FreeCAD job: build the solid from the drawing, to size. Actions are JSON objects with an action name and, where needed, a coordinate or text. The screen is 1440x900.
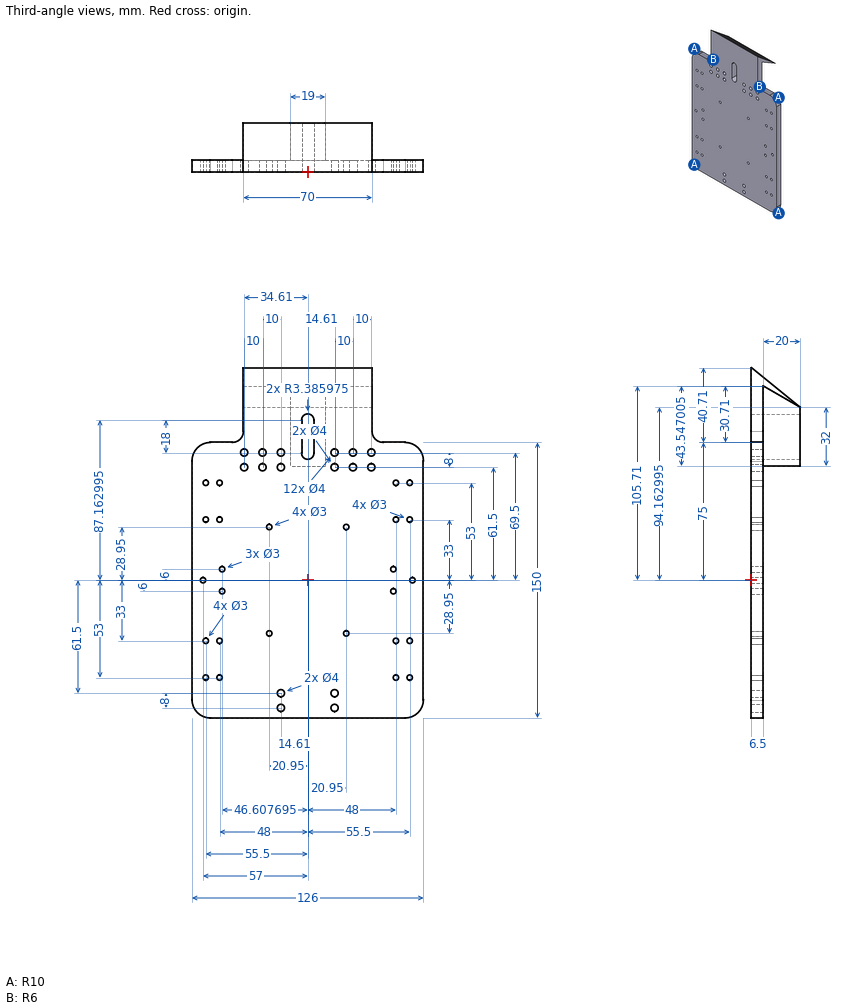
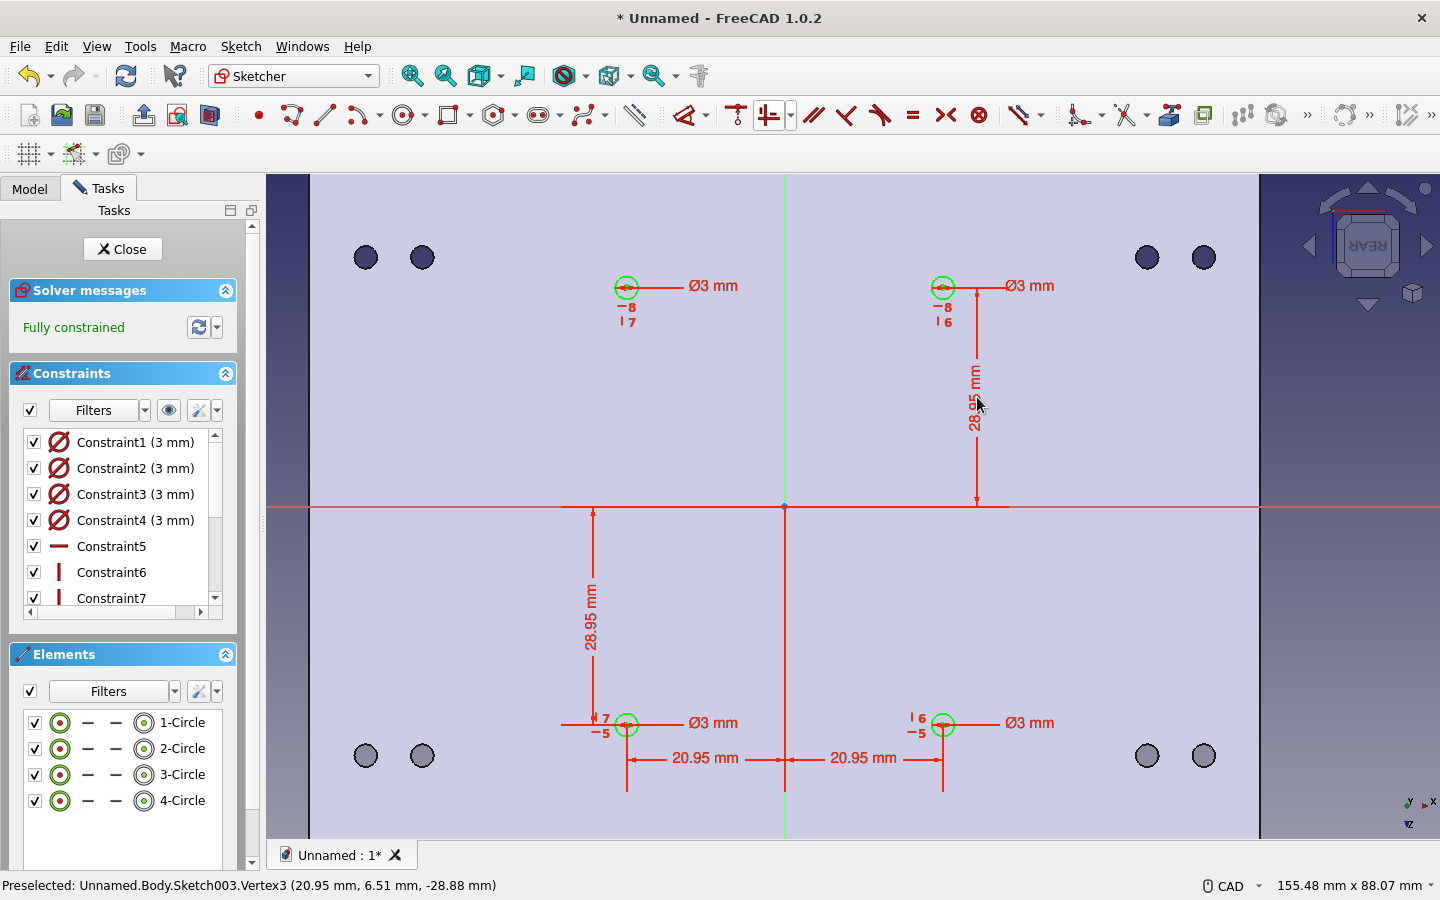
{"action": "left_click", "coordinate": [123, 249]}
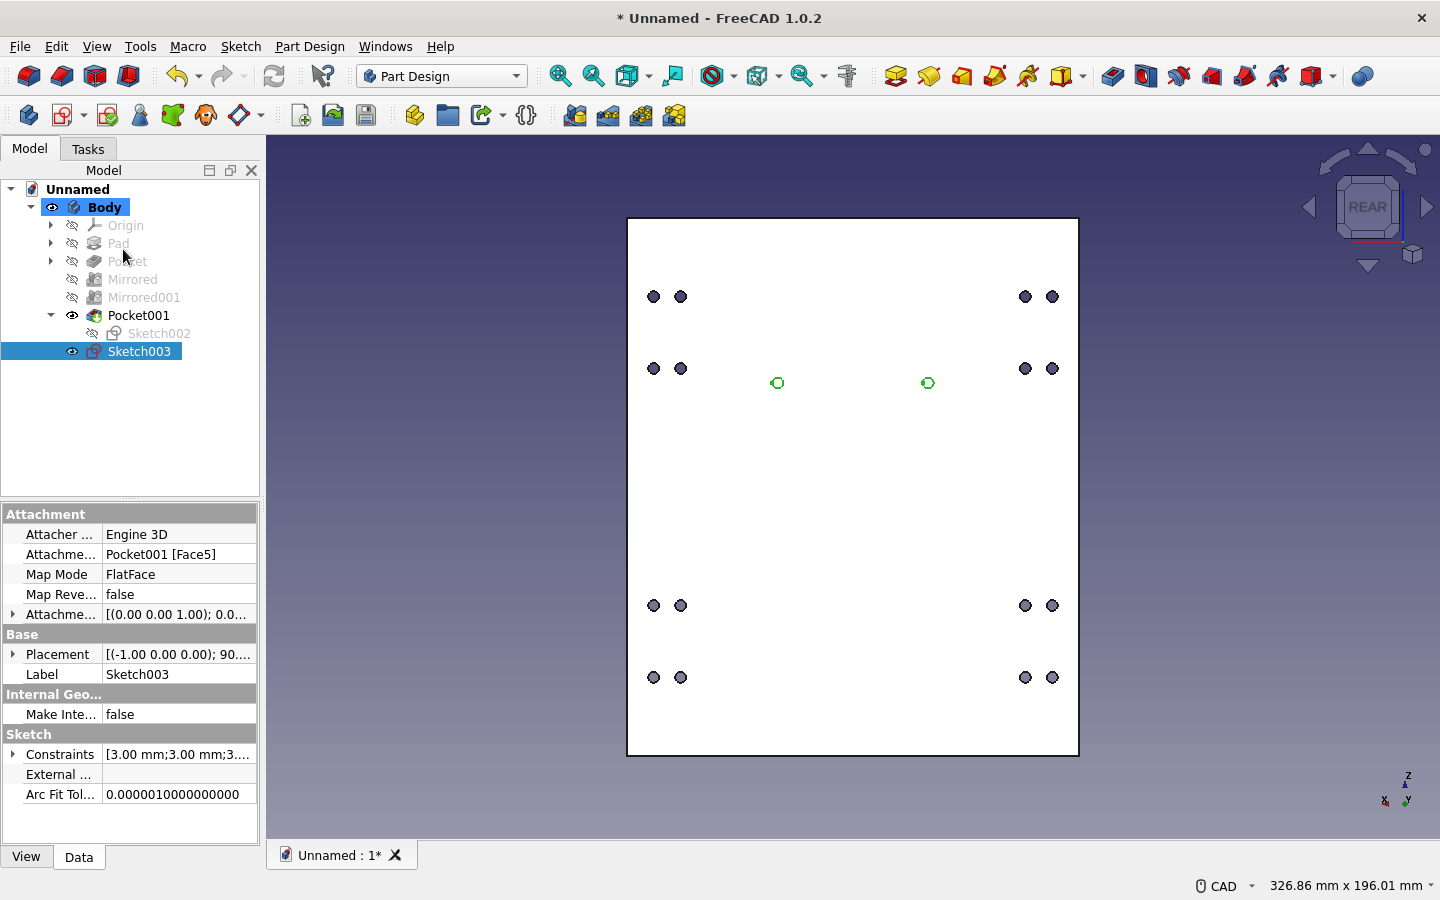
{"action": "left_click", "coordinate": [1113, 76]}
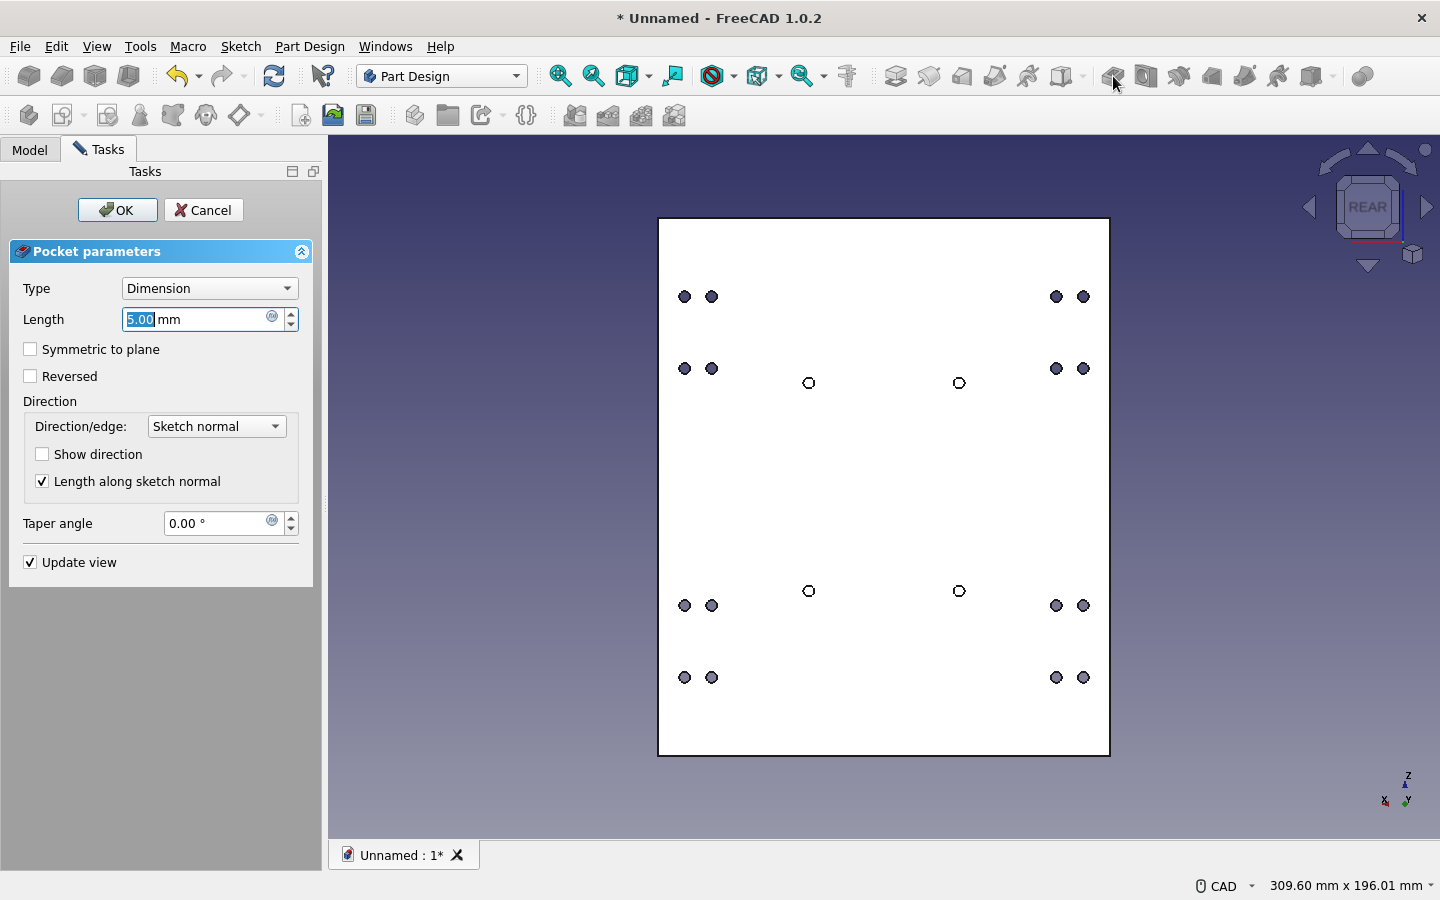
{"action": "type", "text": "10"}
{"action": "key", "text": "Tab"}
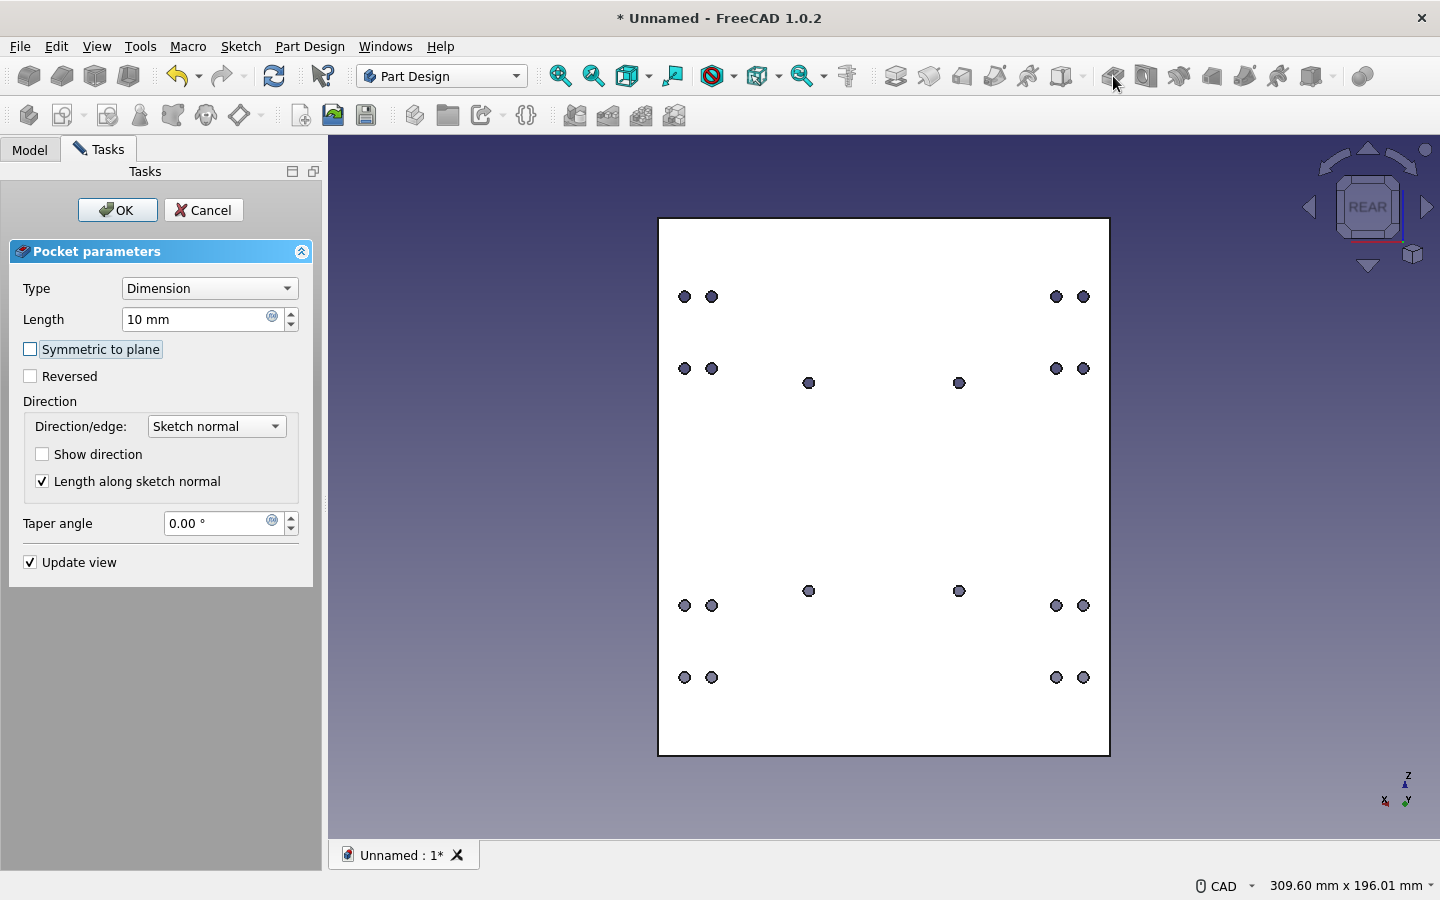
{"action": "left_click", "coordinate": [118, 210]}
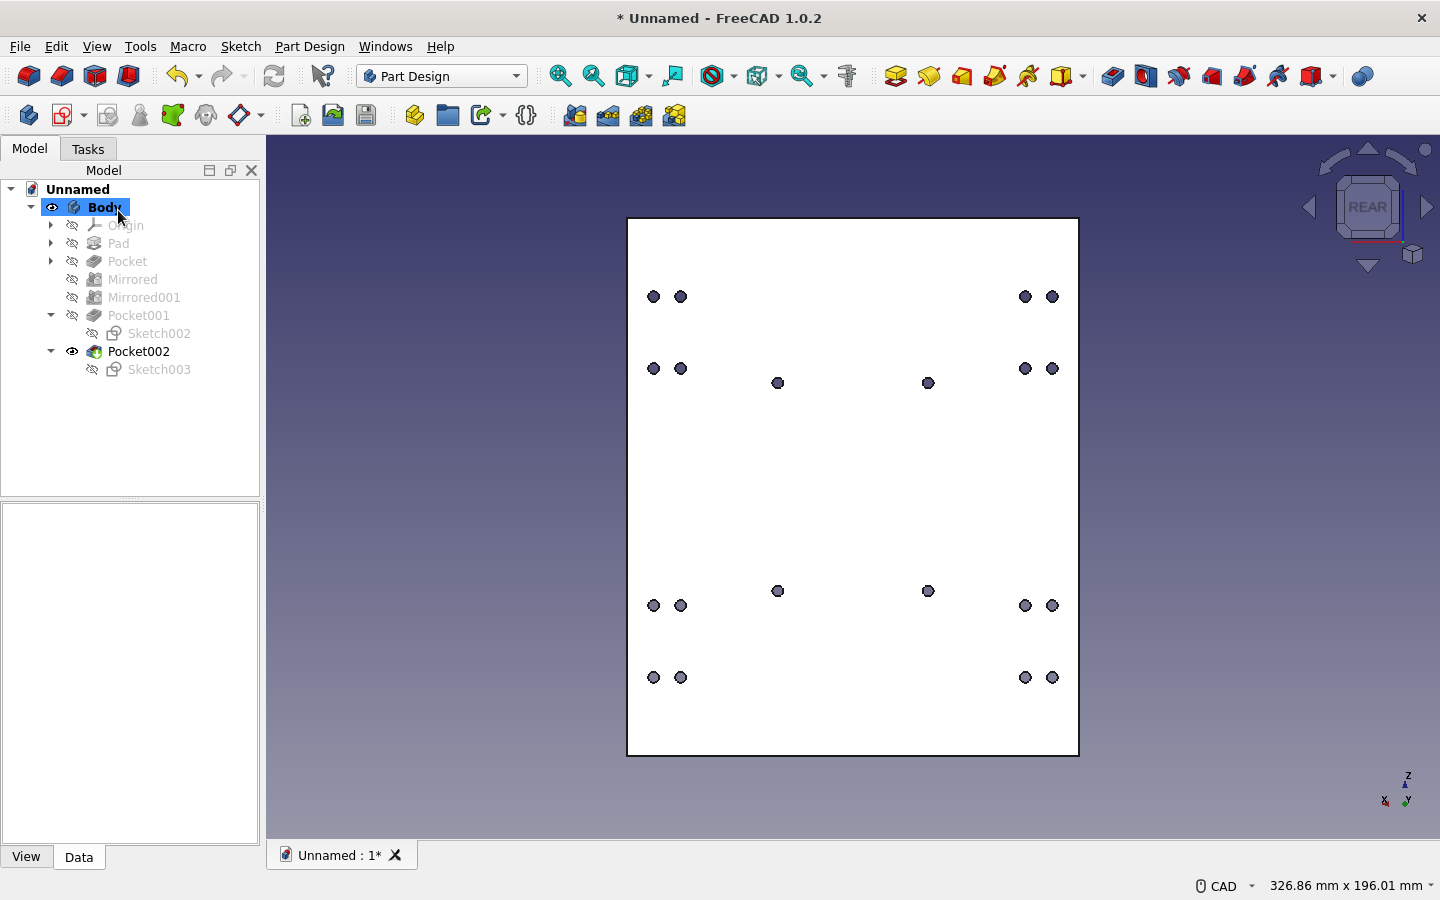
{"action": "key", "text": "0"}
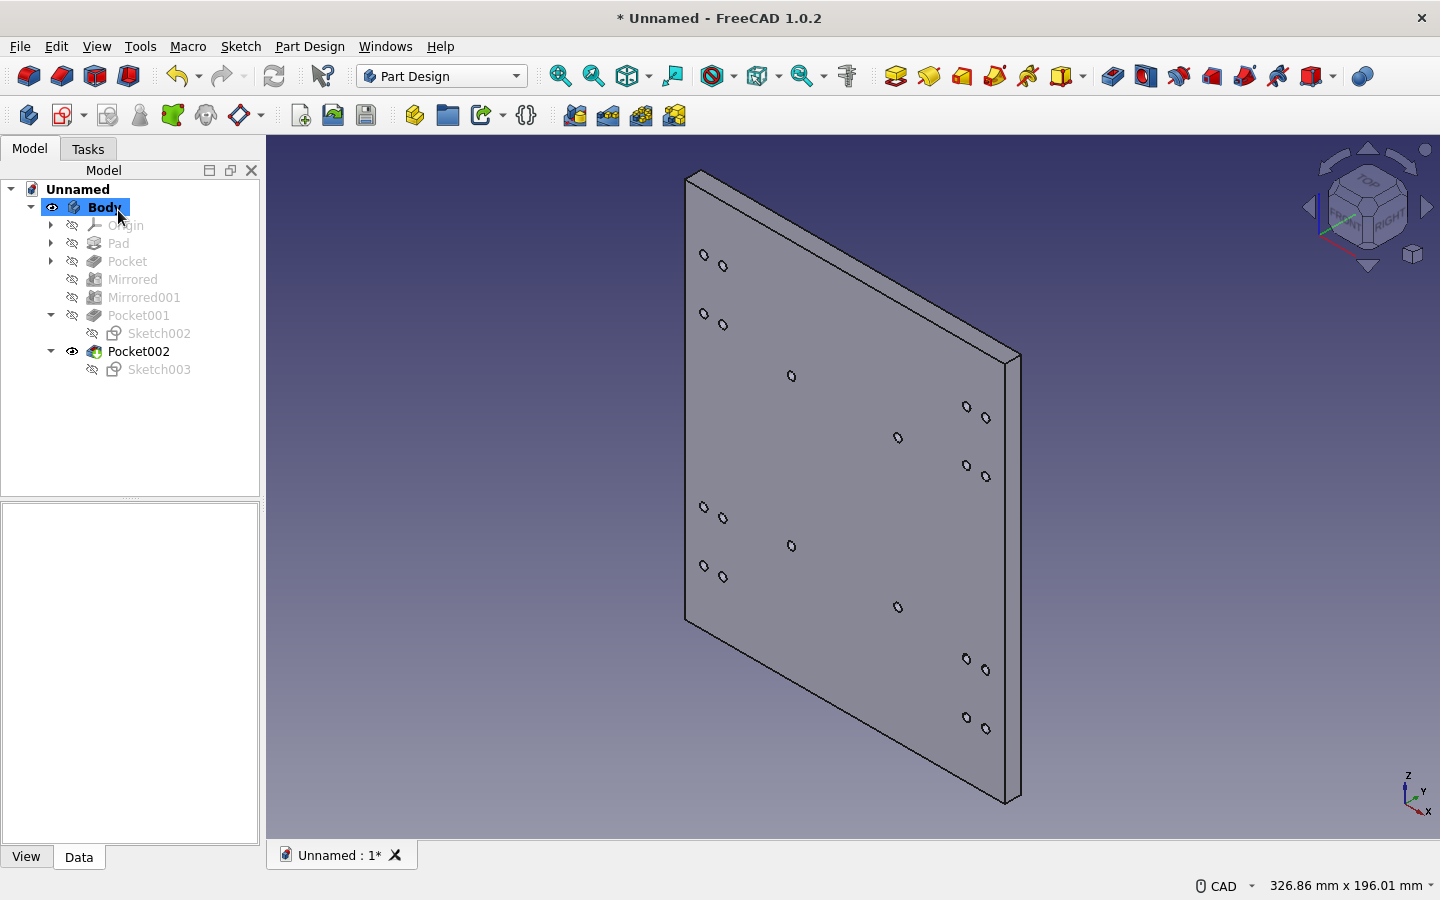
{"action": "left_click", "coordinate": [1013, 358]}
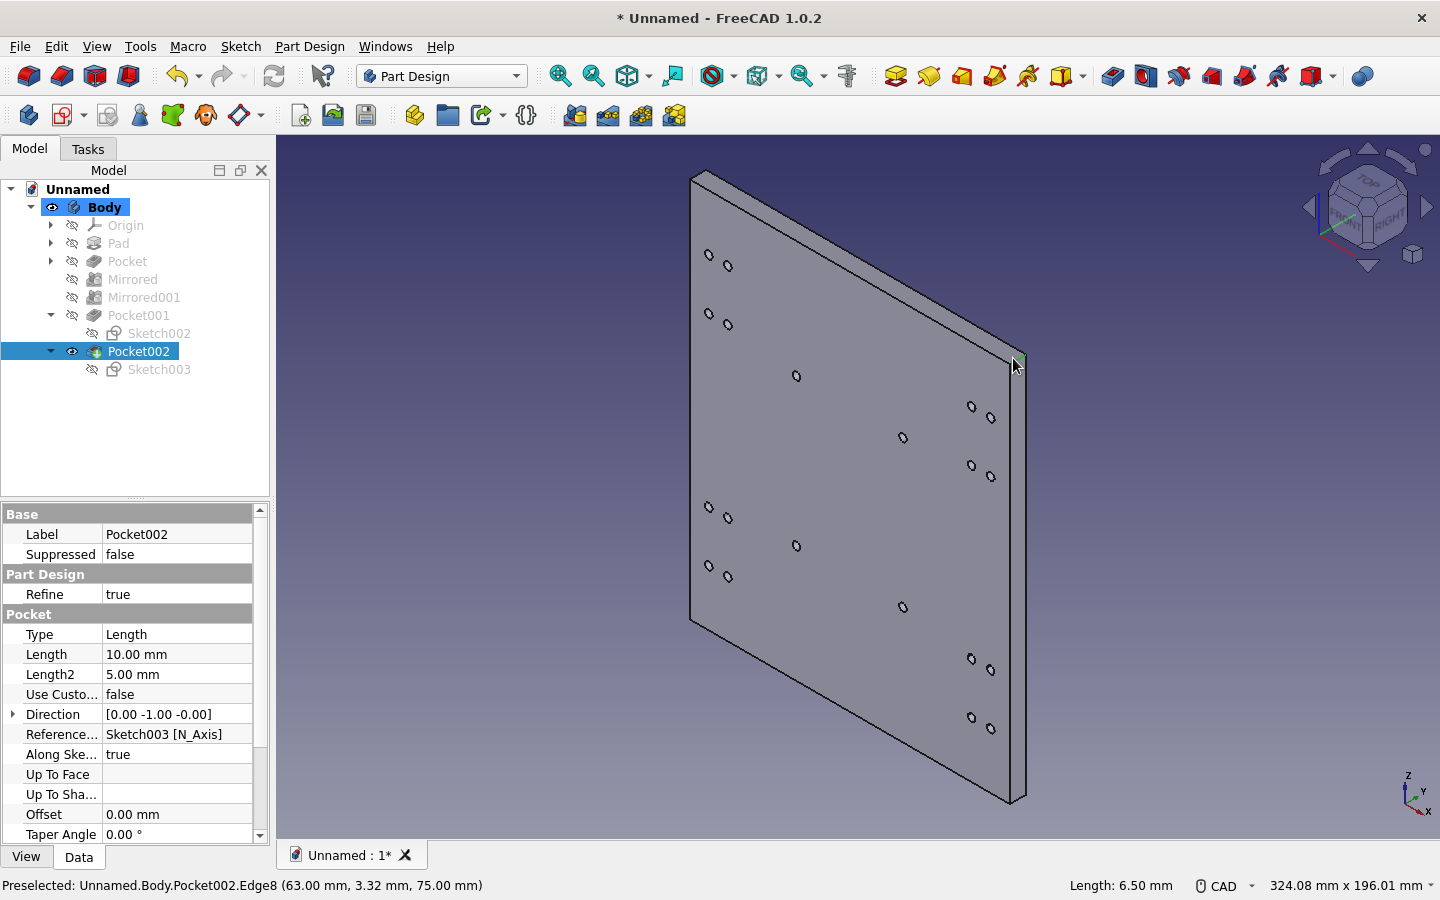
{"action": "key", "text": "2"}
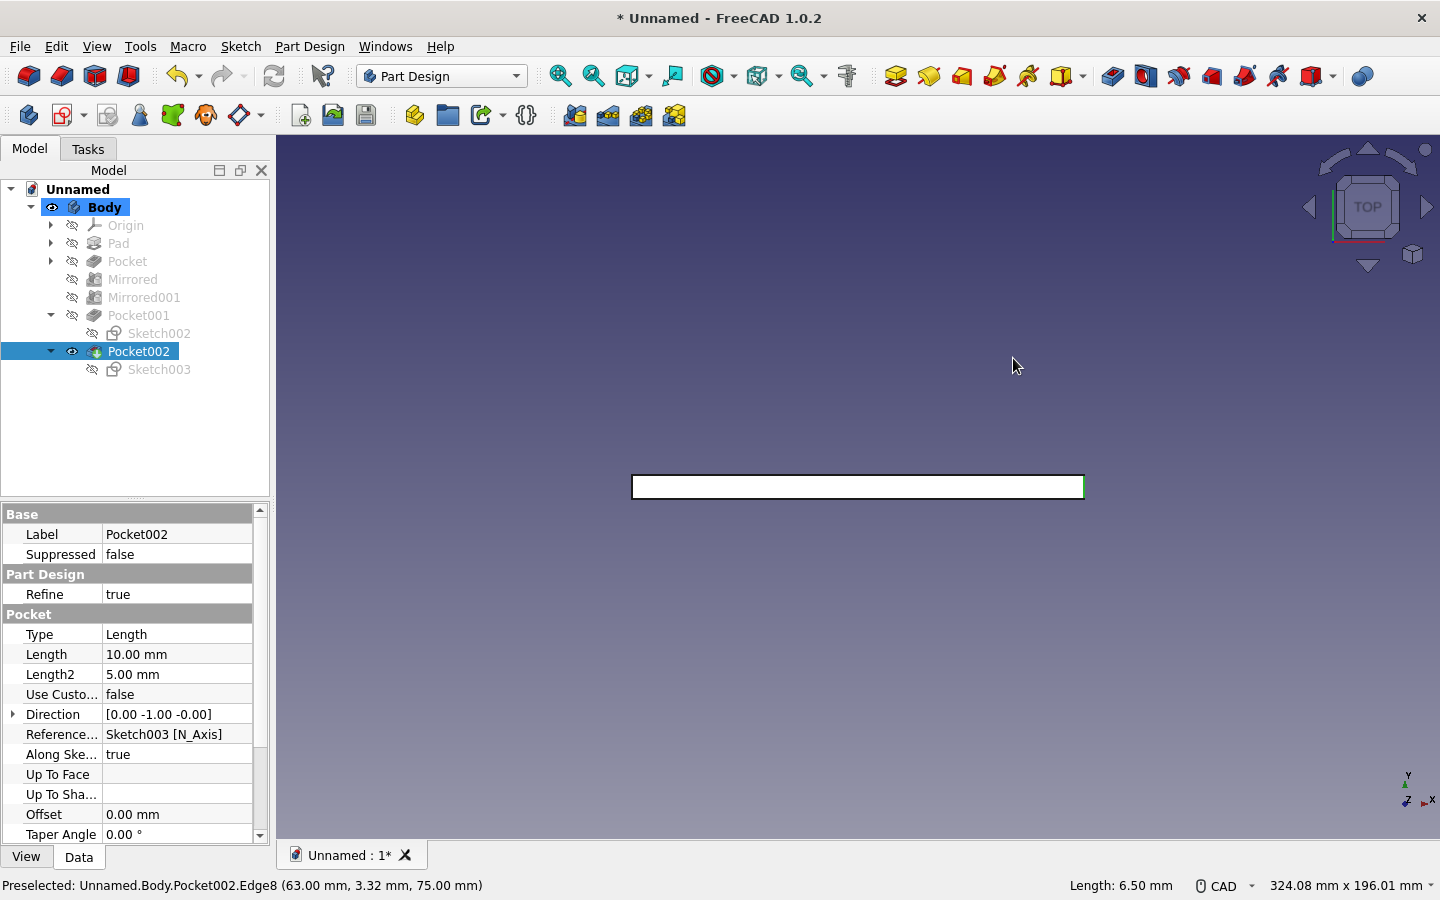
{"action": "left_click", "coordinate": [561, 76]}